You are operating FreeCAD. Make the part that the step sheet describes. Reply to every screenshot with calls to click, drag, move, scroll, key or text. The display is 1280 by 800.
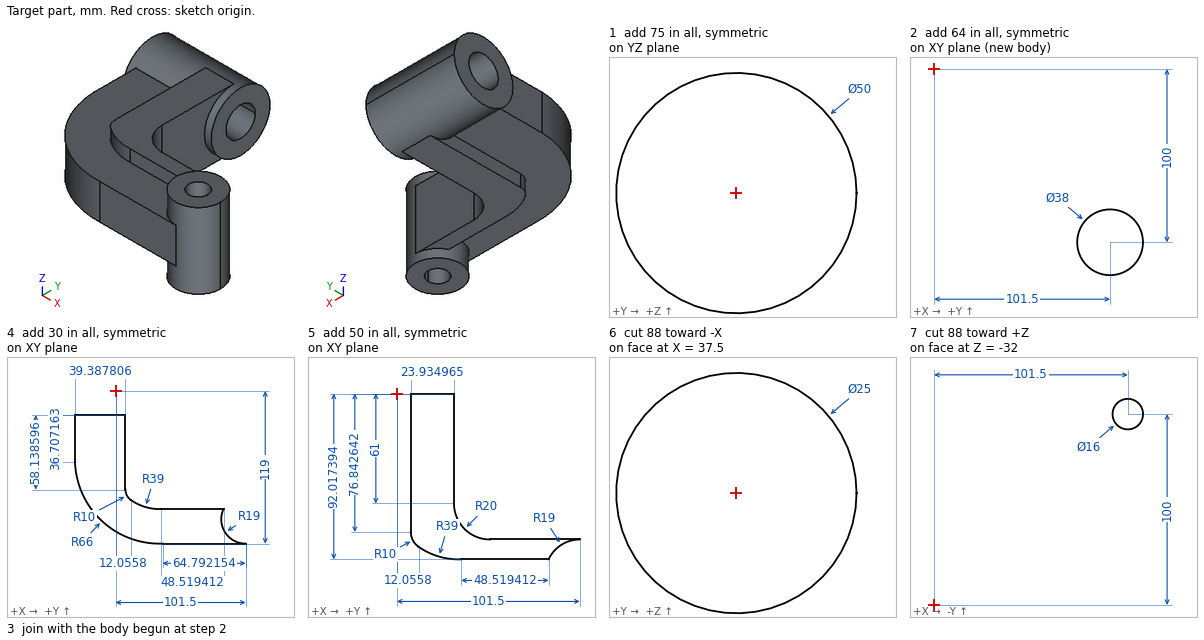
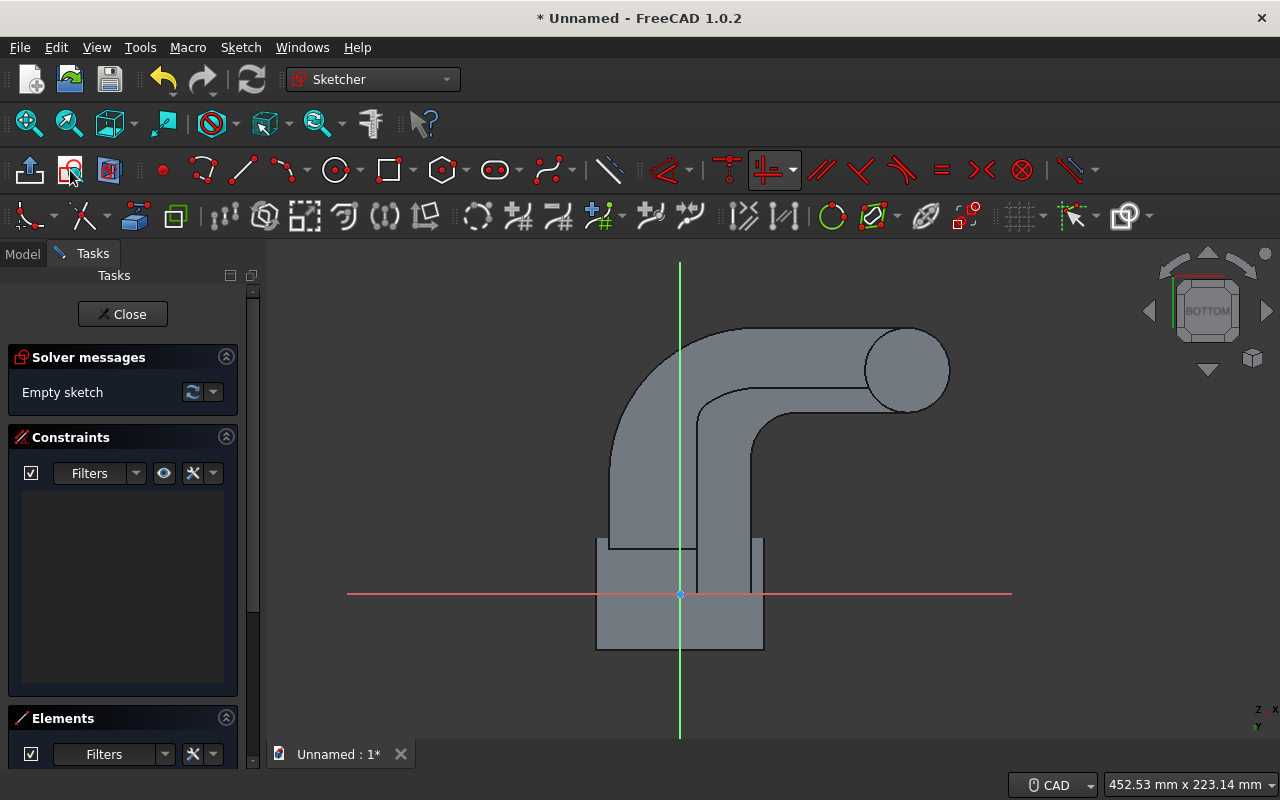
scroll(933, 355, up, 11)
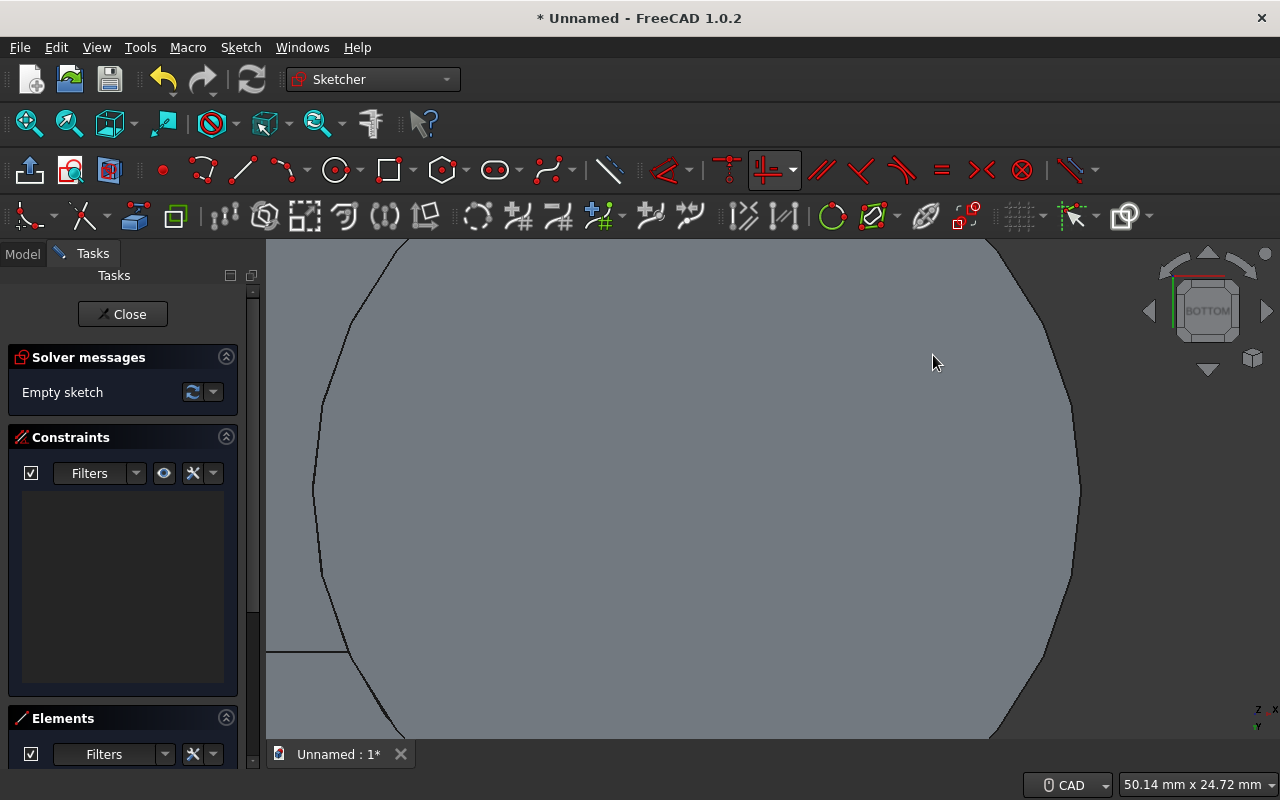
click(336, 170)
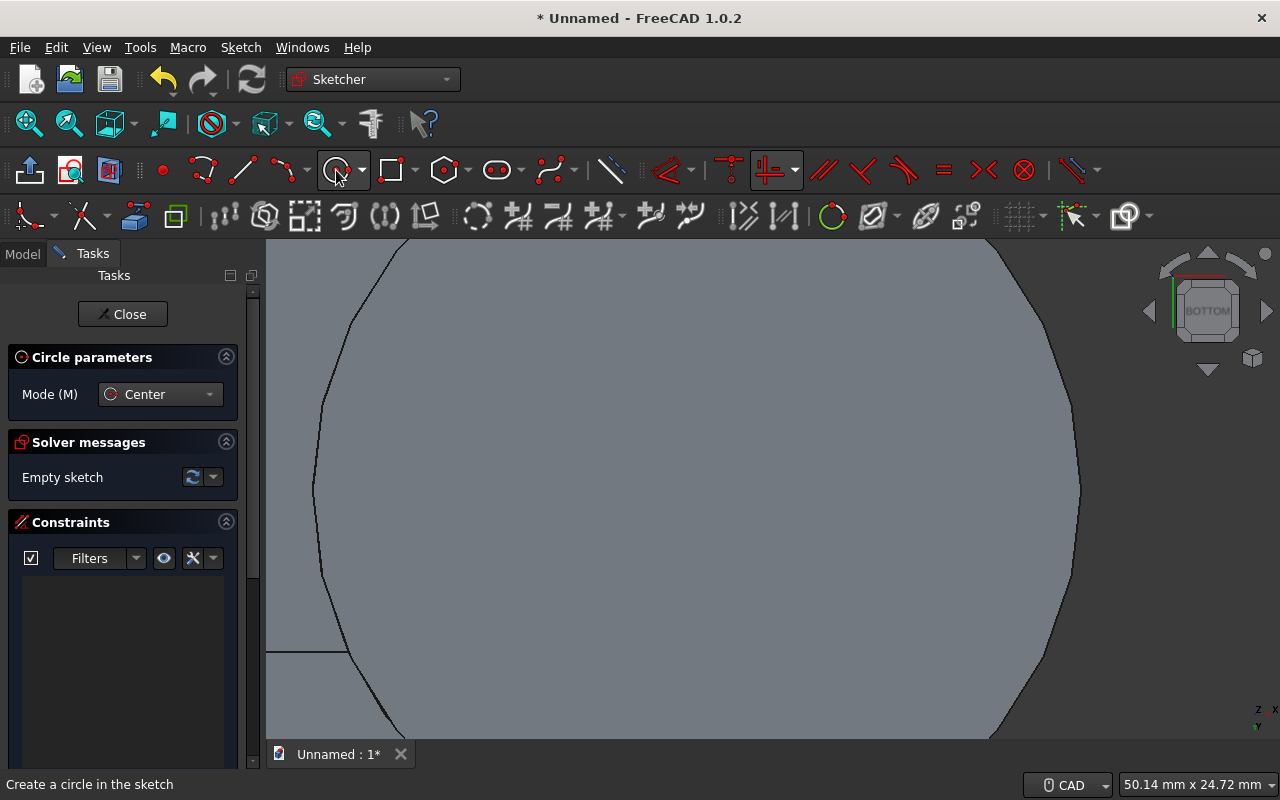
click(697, 491)
click(811, 376)
key(Escape)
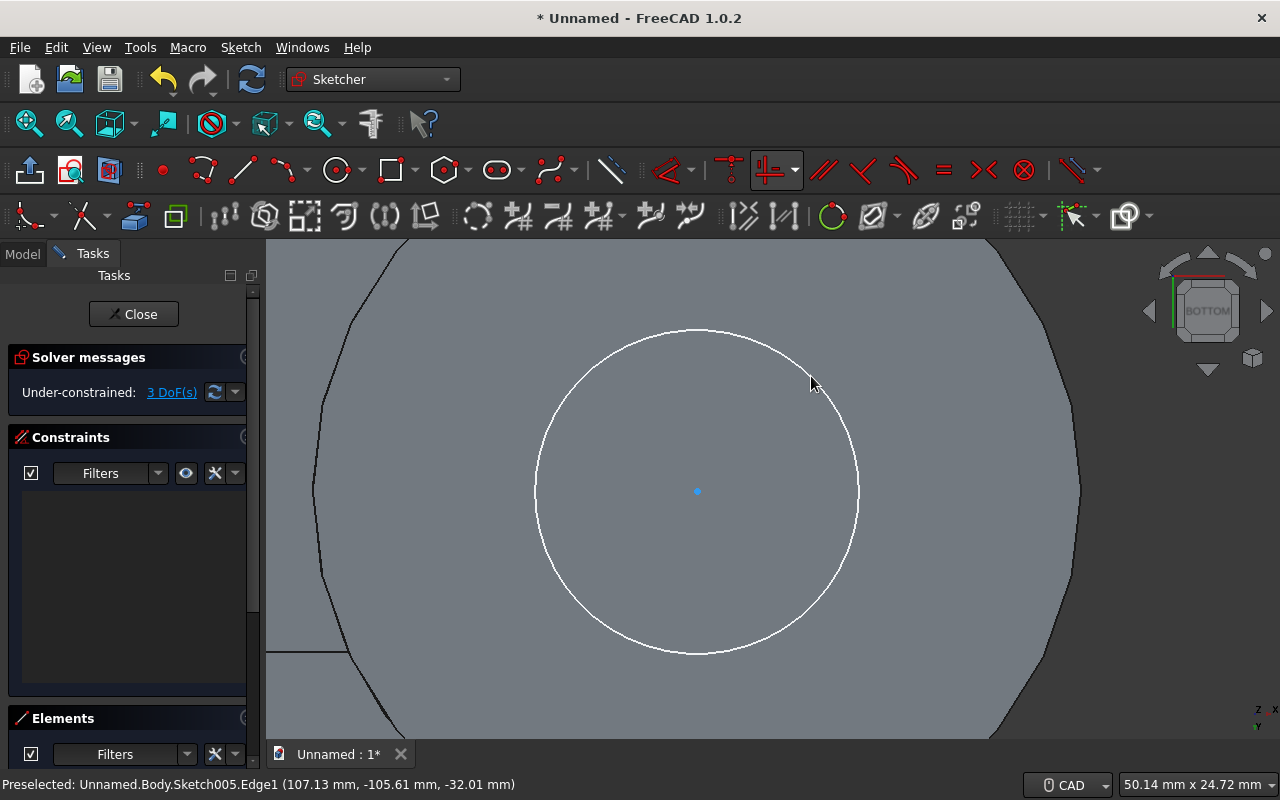
click(666, 170)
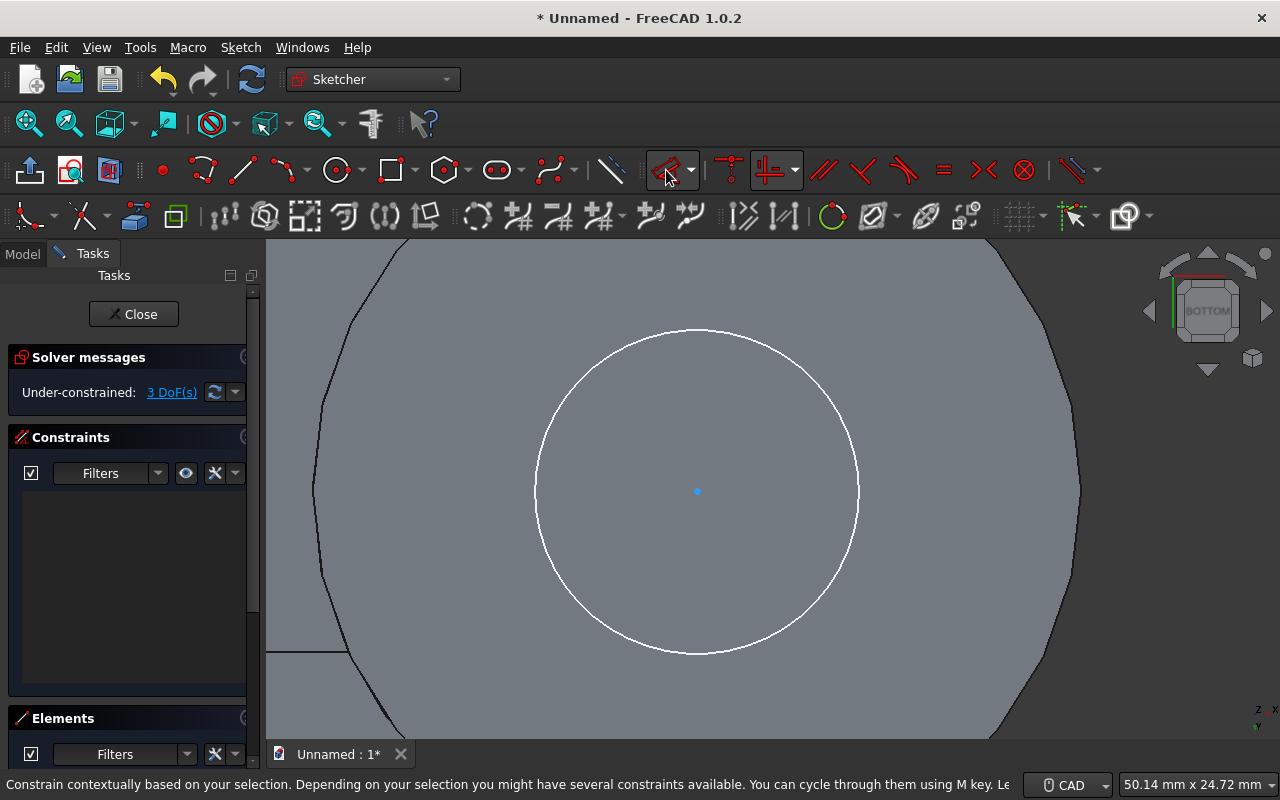
click(811, 377)
click(834, 354)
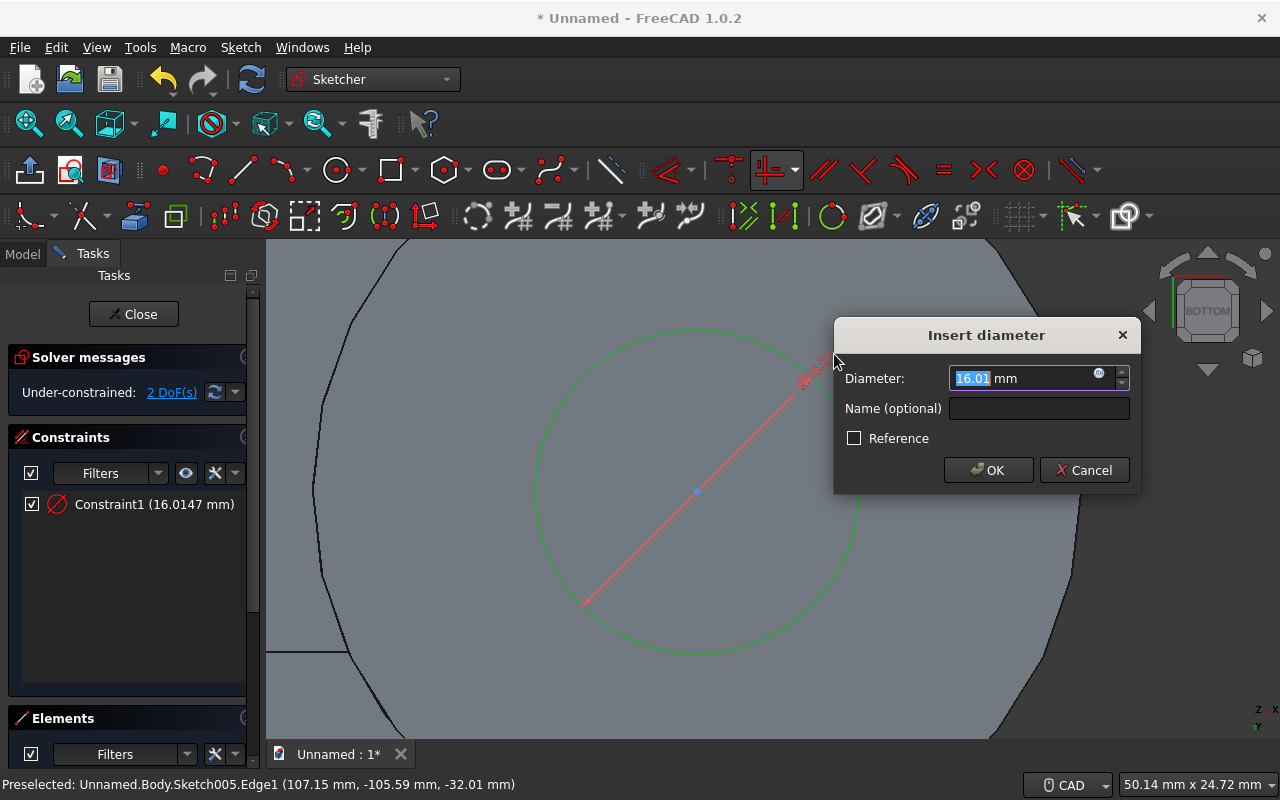
text(16)
key(Return)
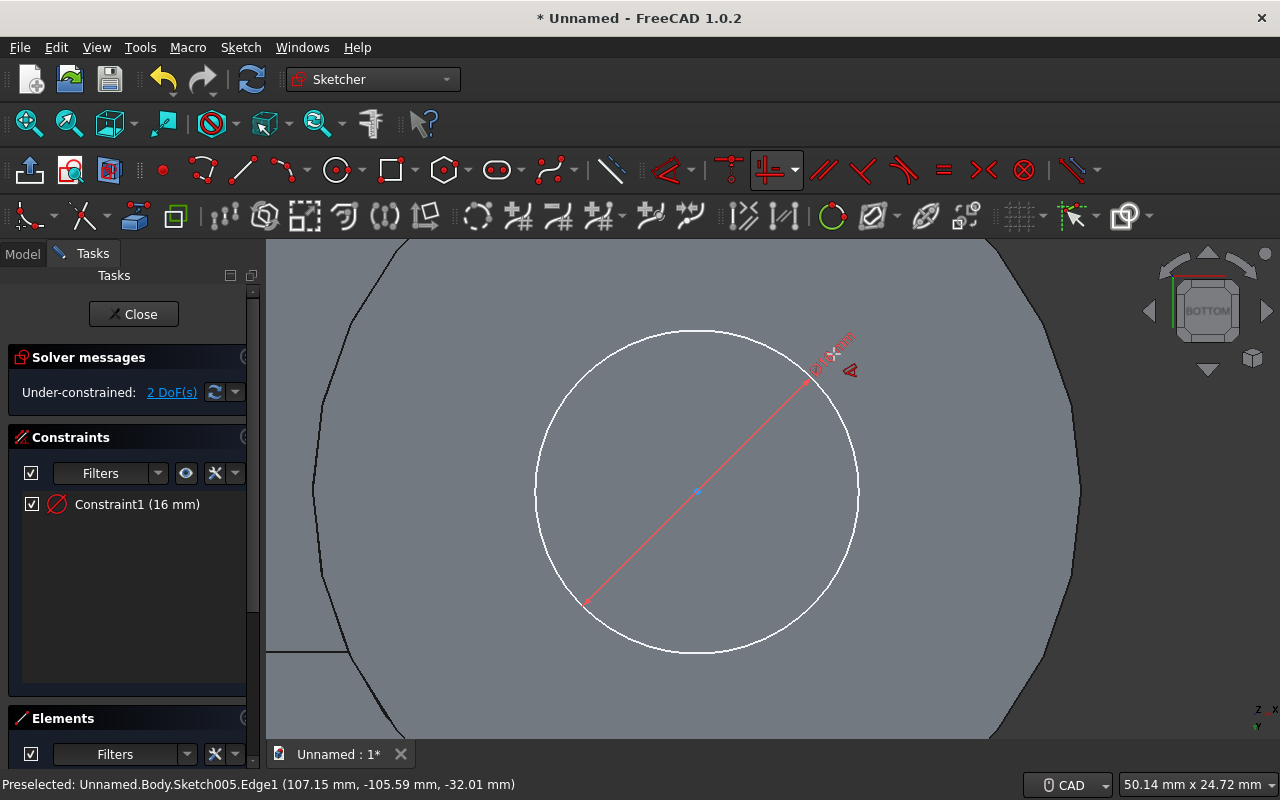
click(697, 492)
click(731, 602)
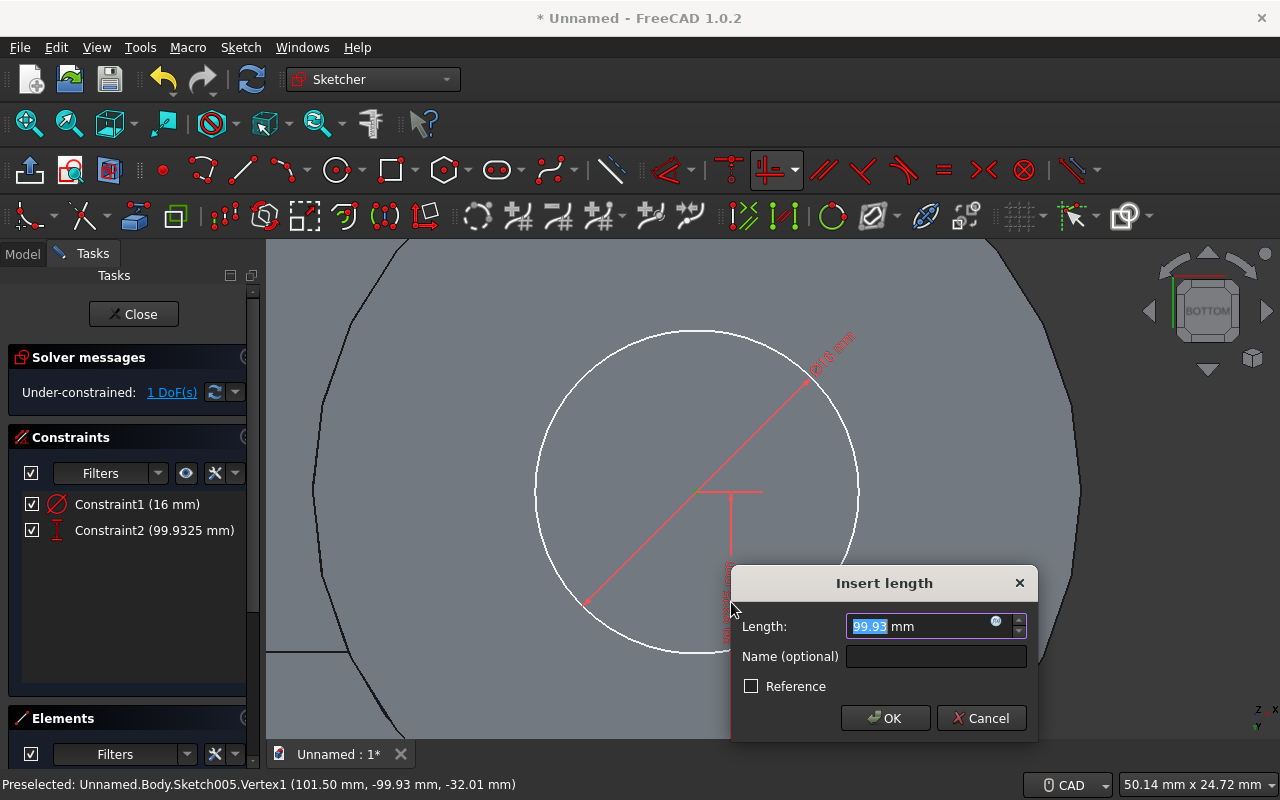
text(100)
key(Return)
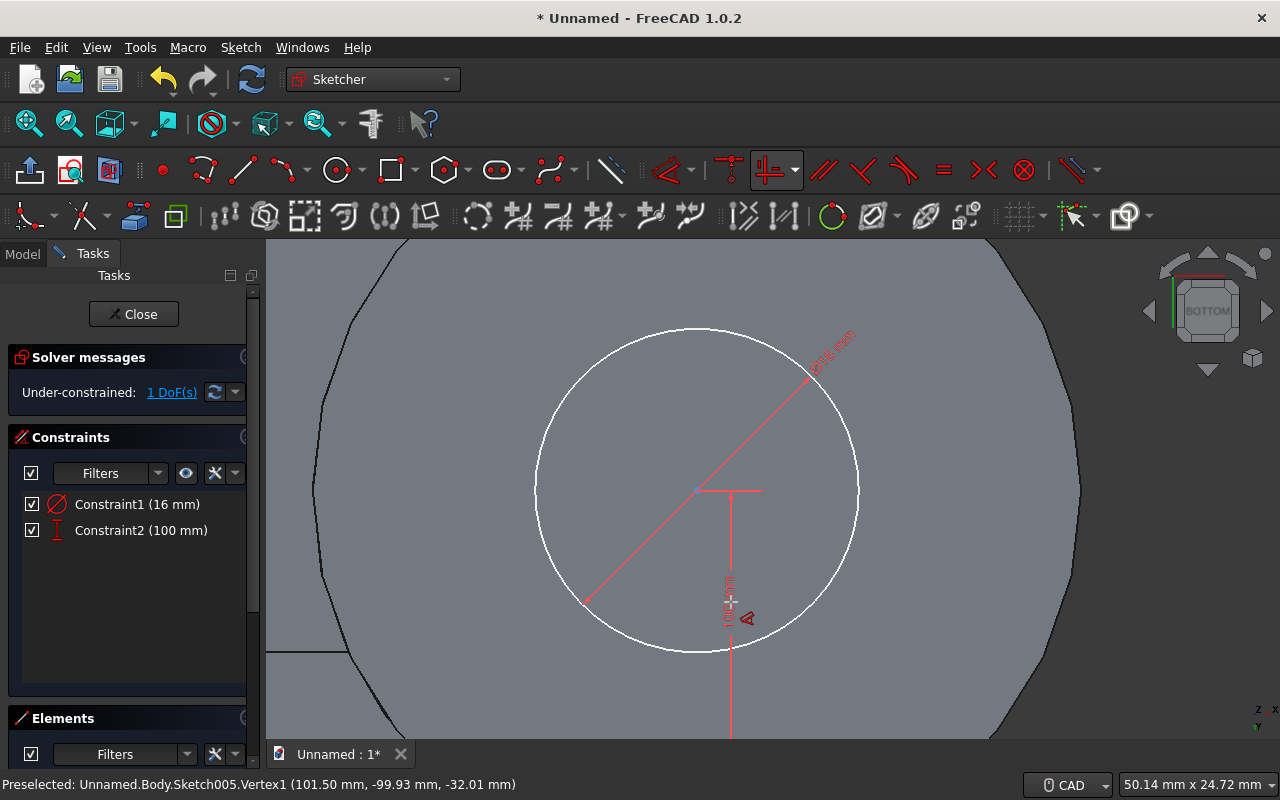
click(697, 491)
click(496, 457)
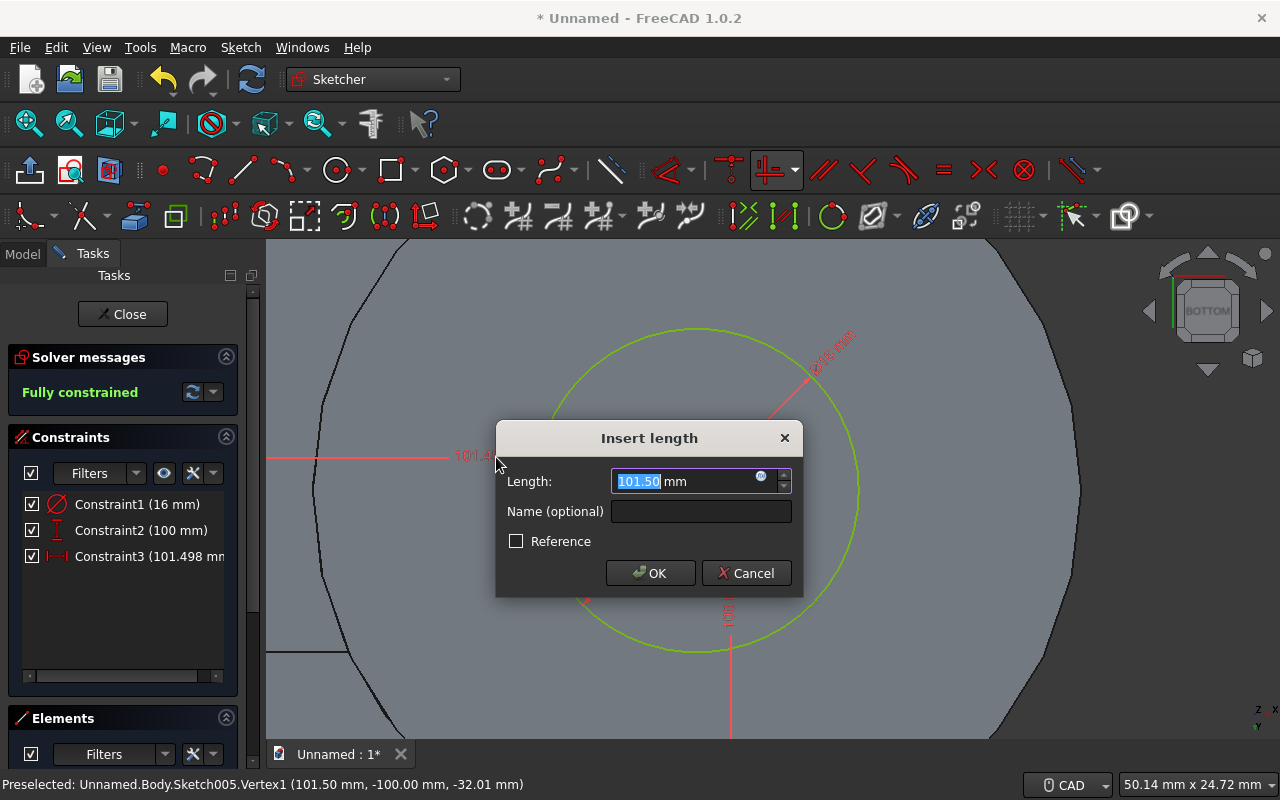
text(101.5)
key(Return)
key(Escape)